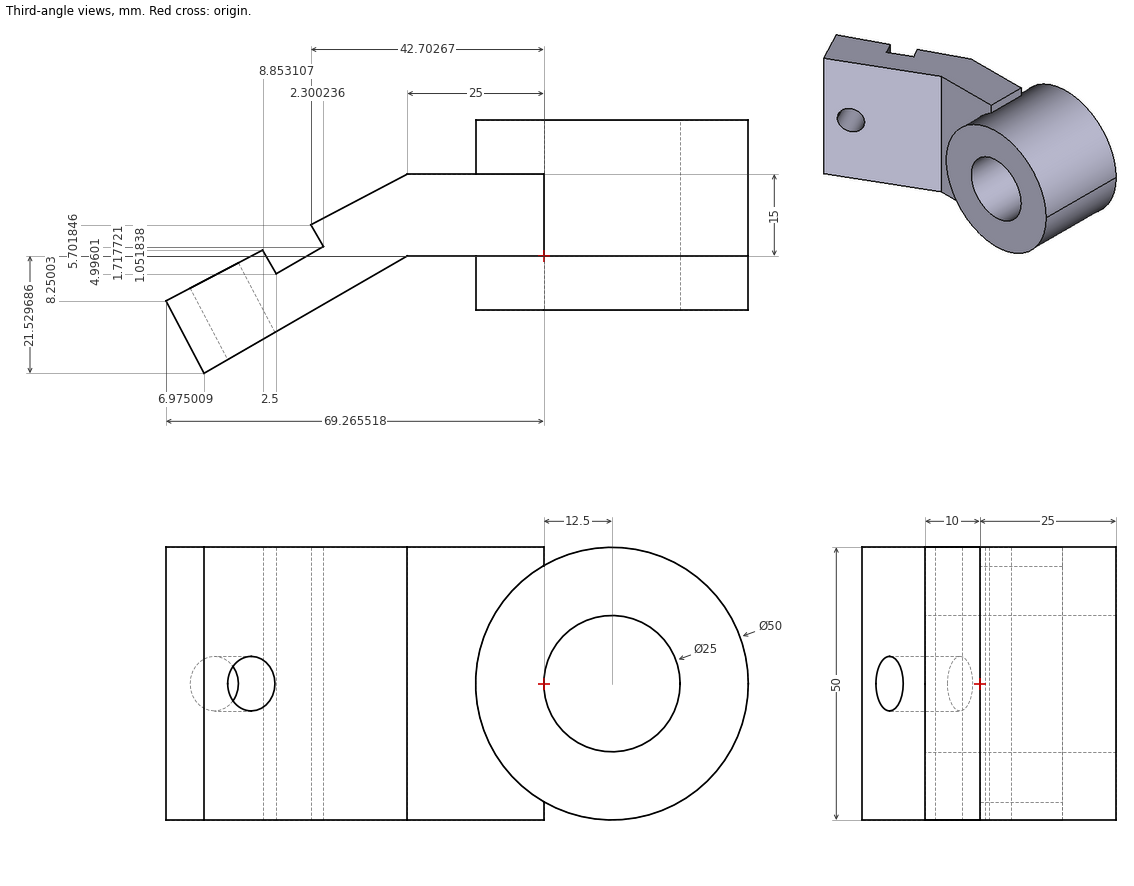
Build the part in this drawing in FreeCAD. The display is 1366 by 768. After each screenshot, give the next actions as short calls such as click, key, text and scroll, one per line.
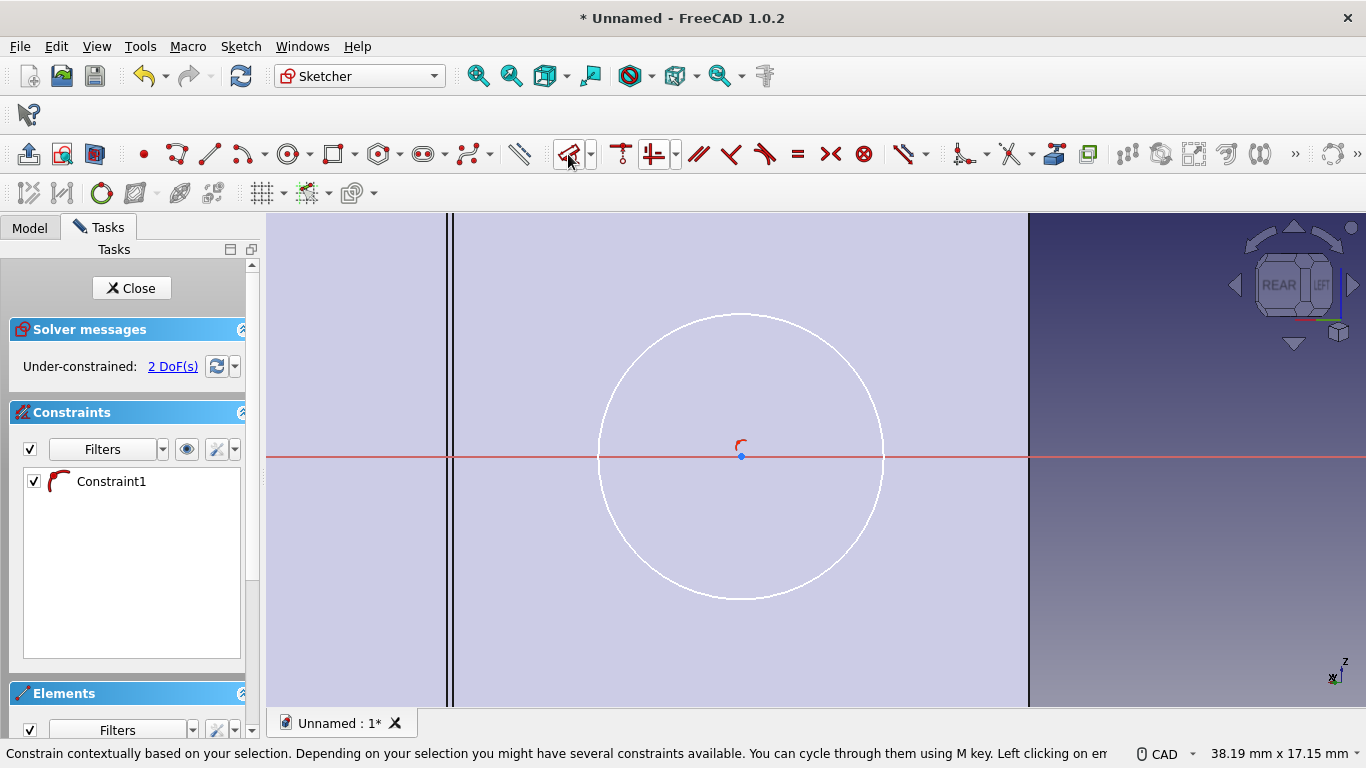
click(842, 356)
click(865, 333)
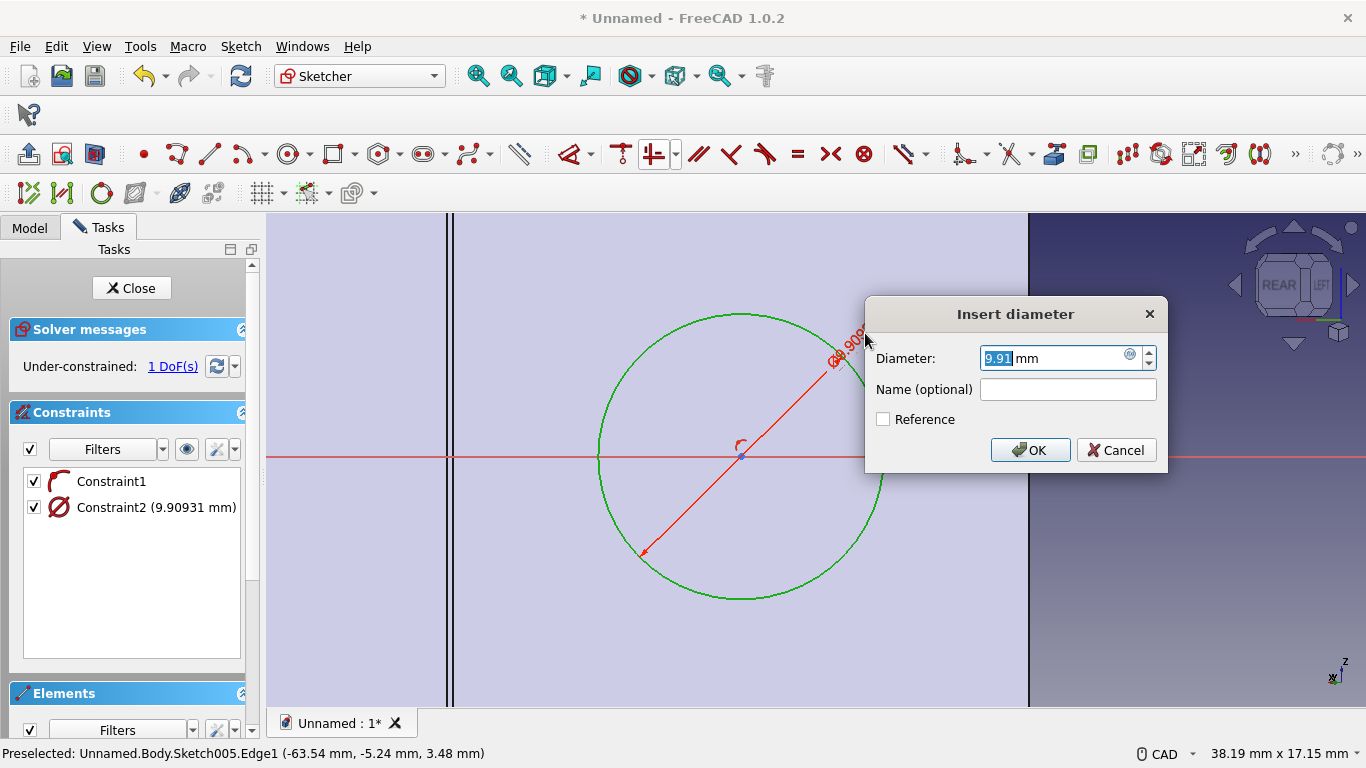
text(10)
key(Return)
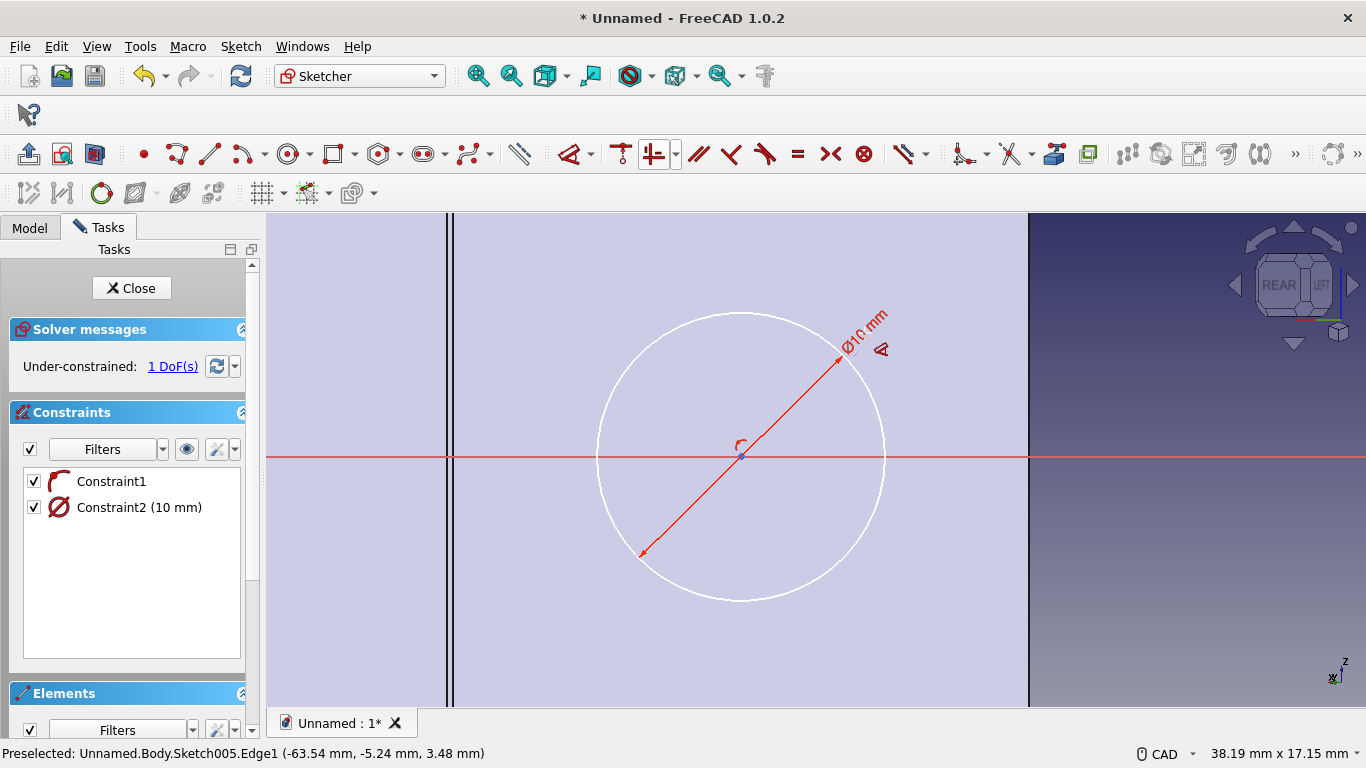
click(741, 457)
click(518, 491)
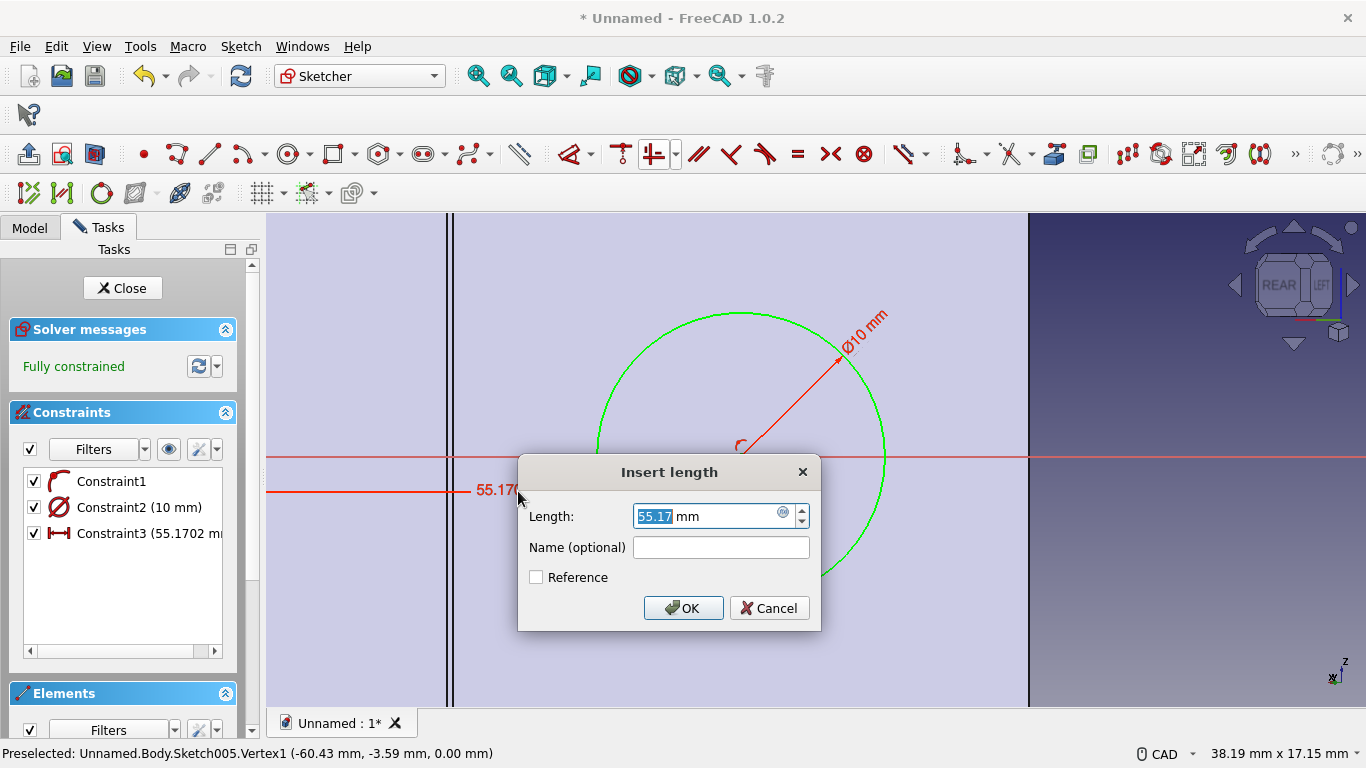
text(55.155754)
key(Return)
key(Escape)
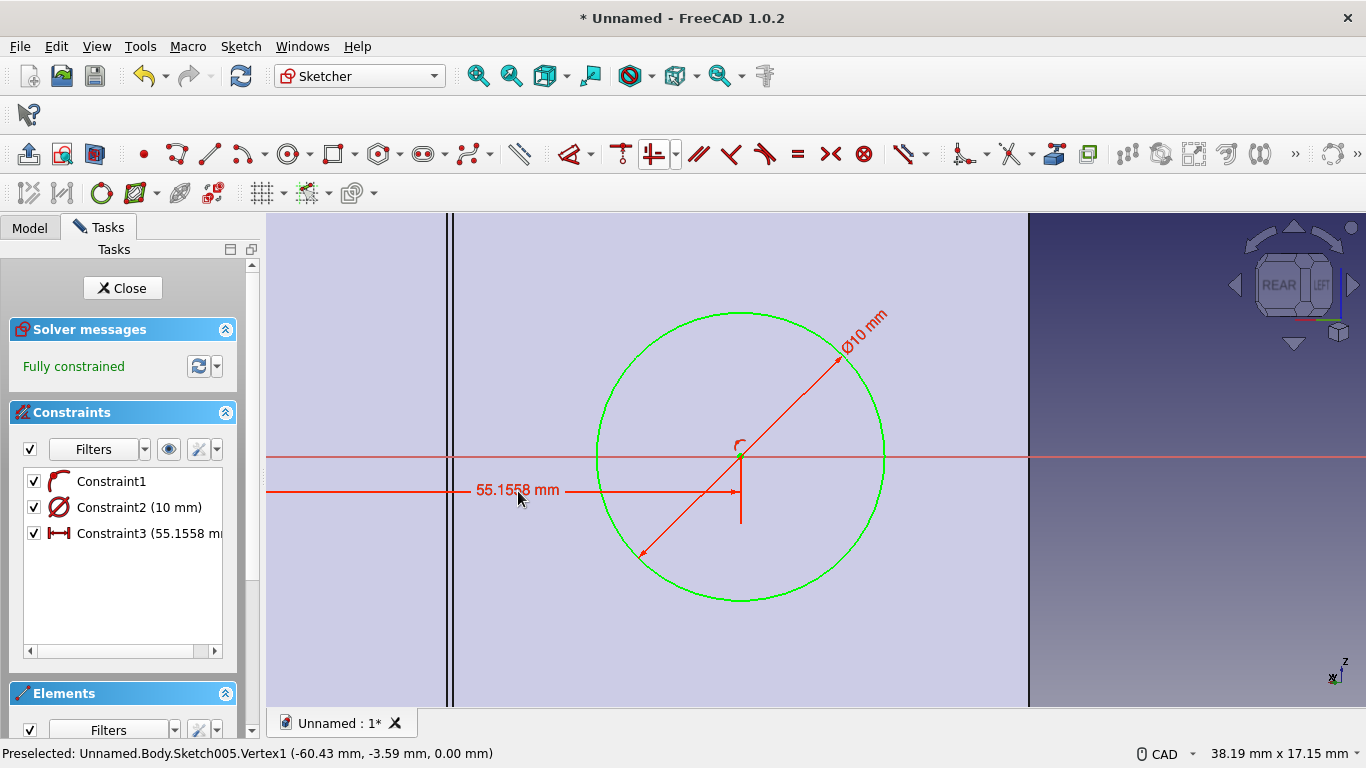
click(123, 288)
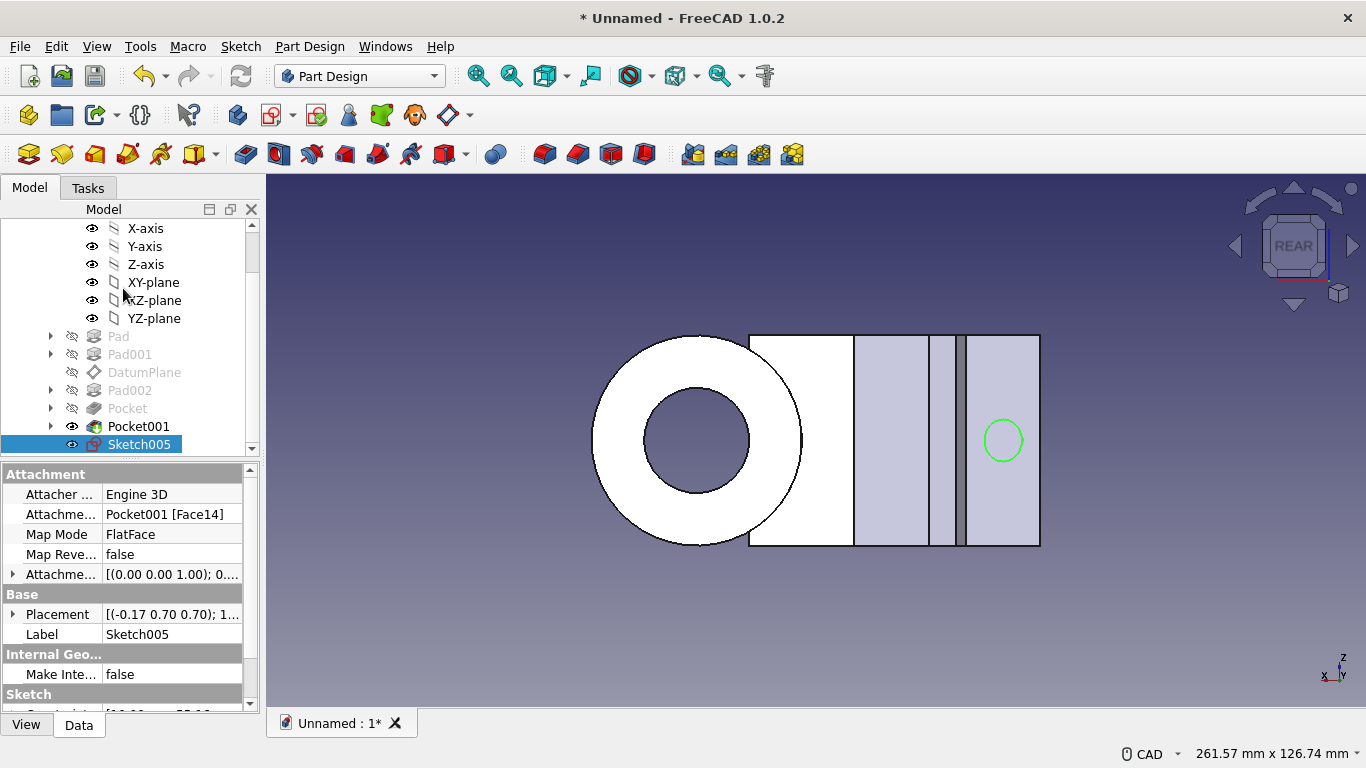
click(246, 154)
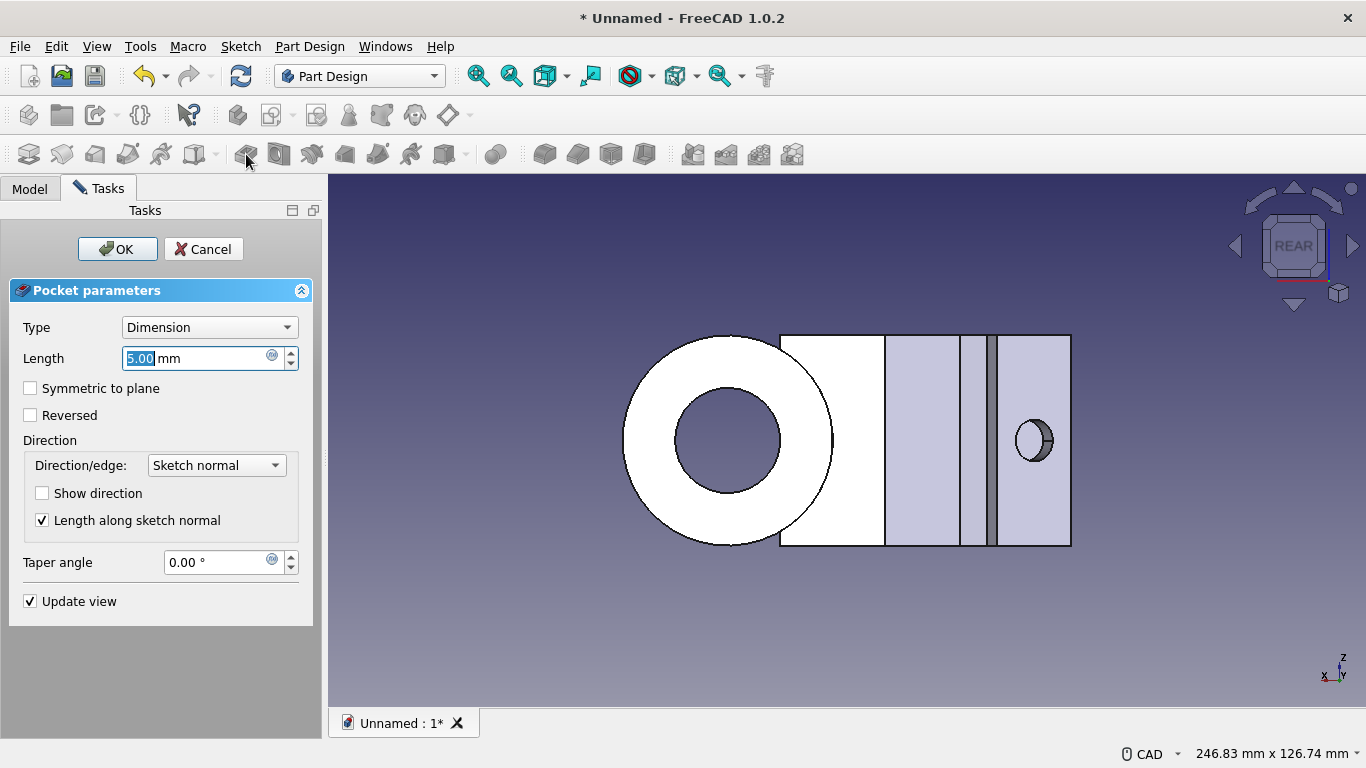
click(210, 328)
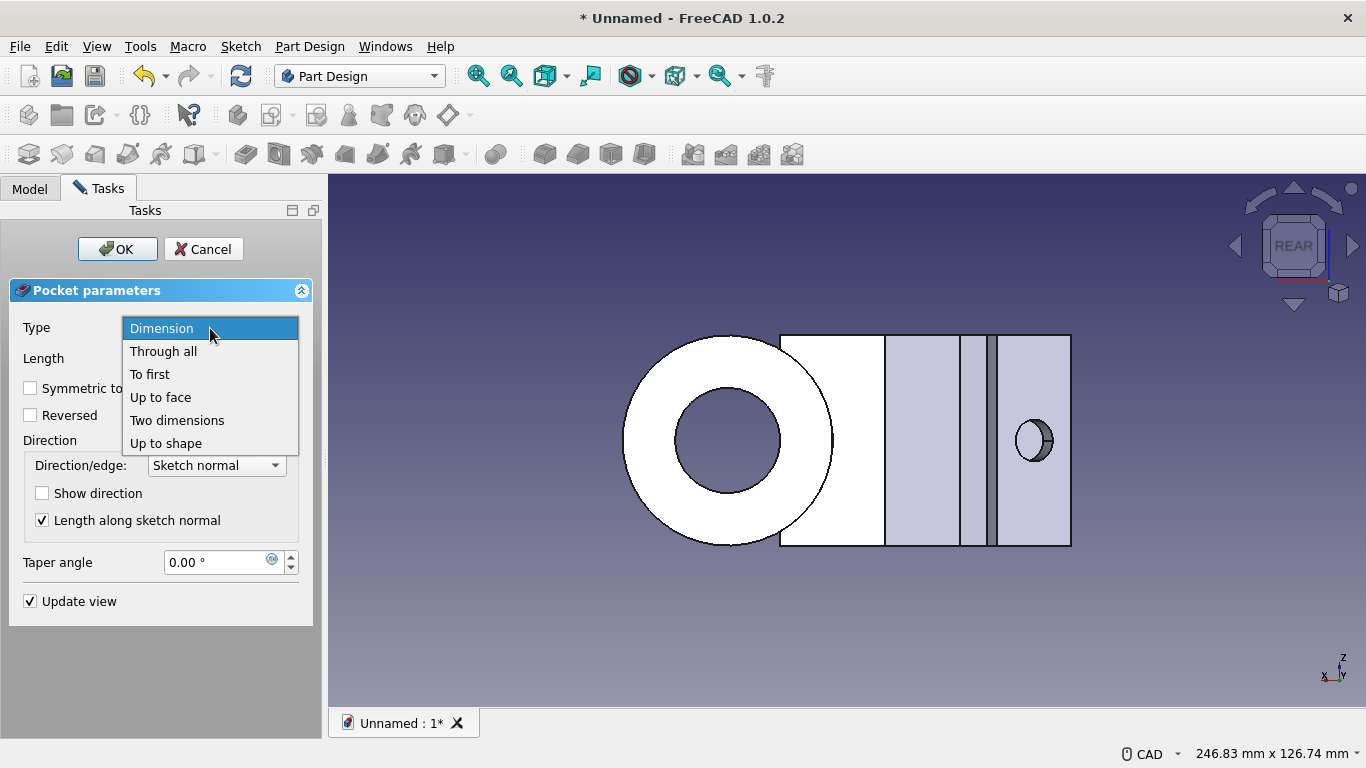
click(208, 352)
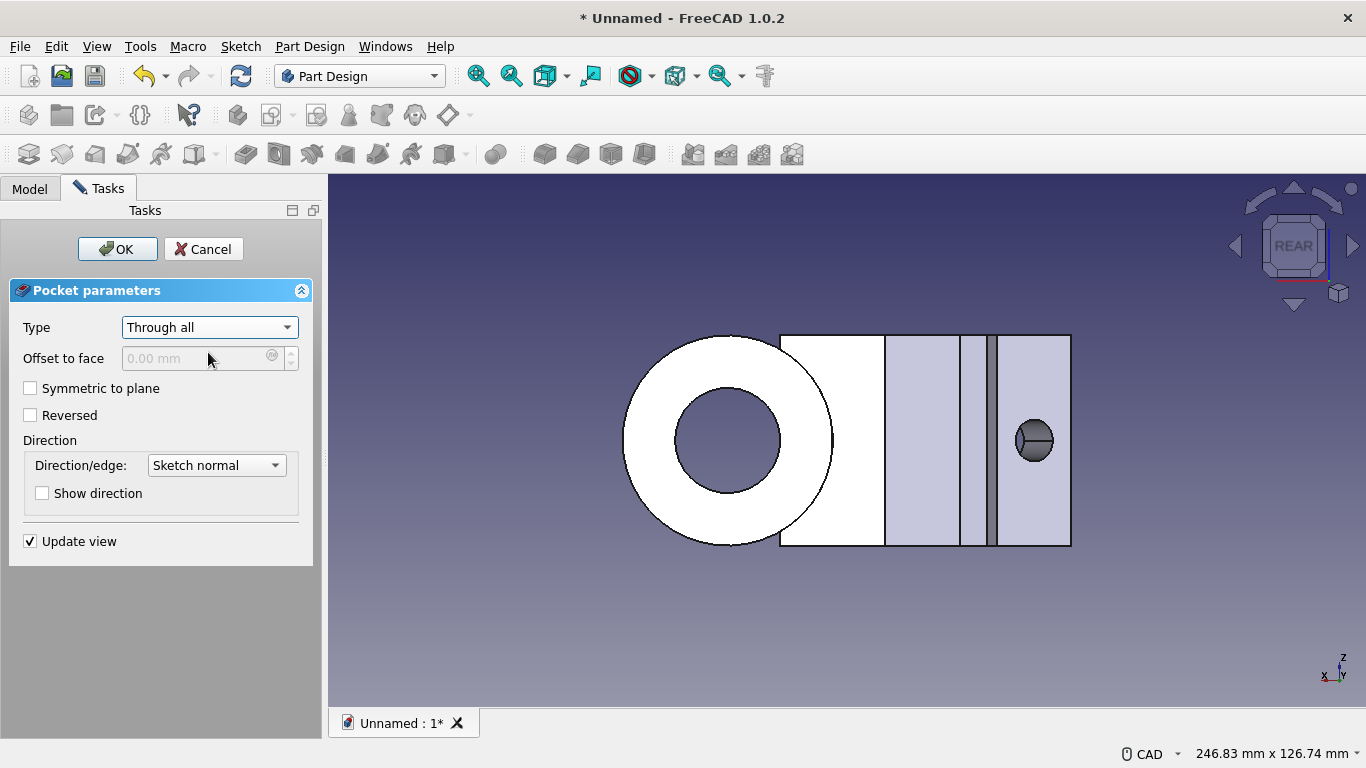
click(118, 249)